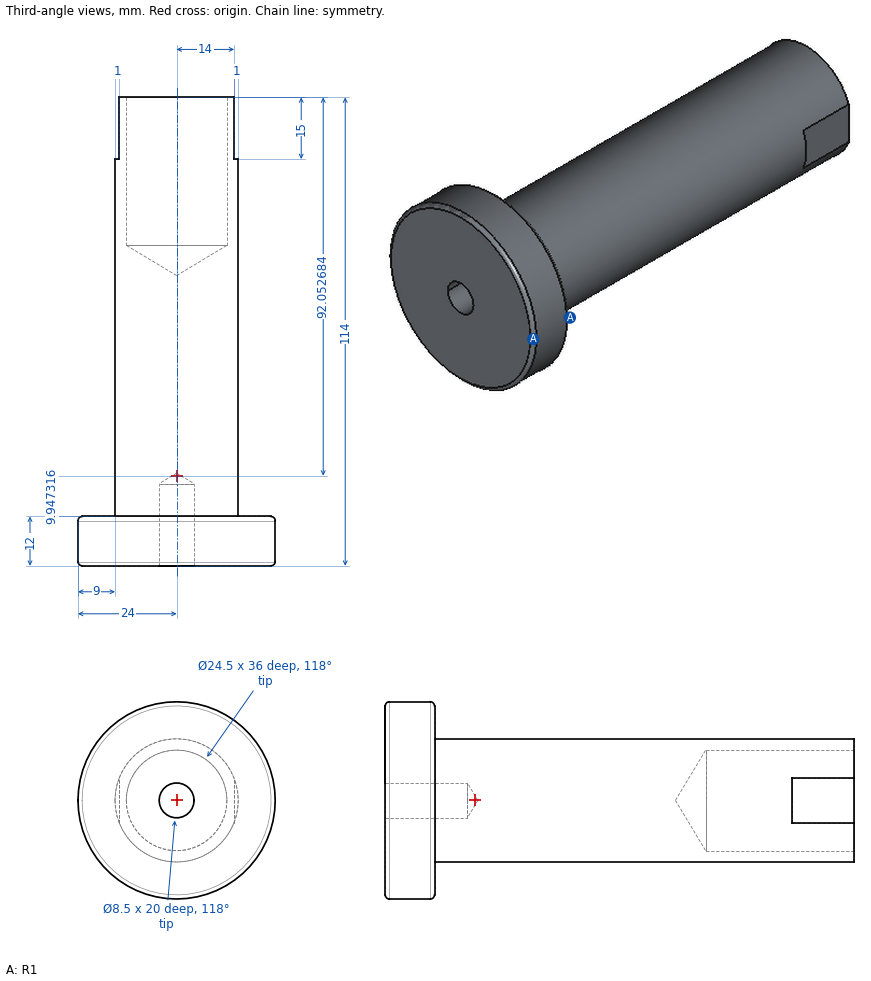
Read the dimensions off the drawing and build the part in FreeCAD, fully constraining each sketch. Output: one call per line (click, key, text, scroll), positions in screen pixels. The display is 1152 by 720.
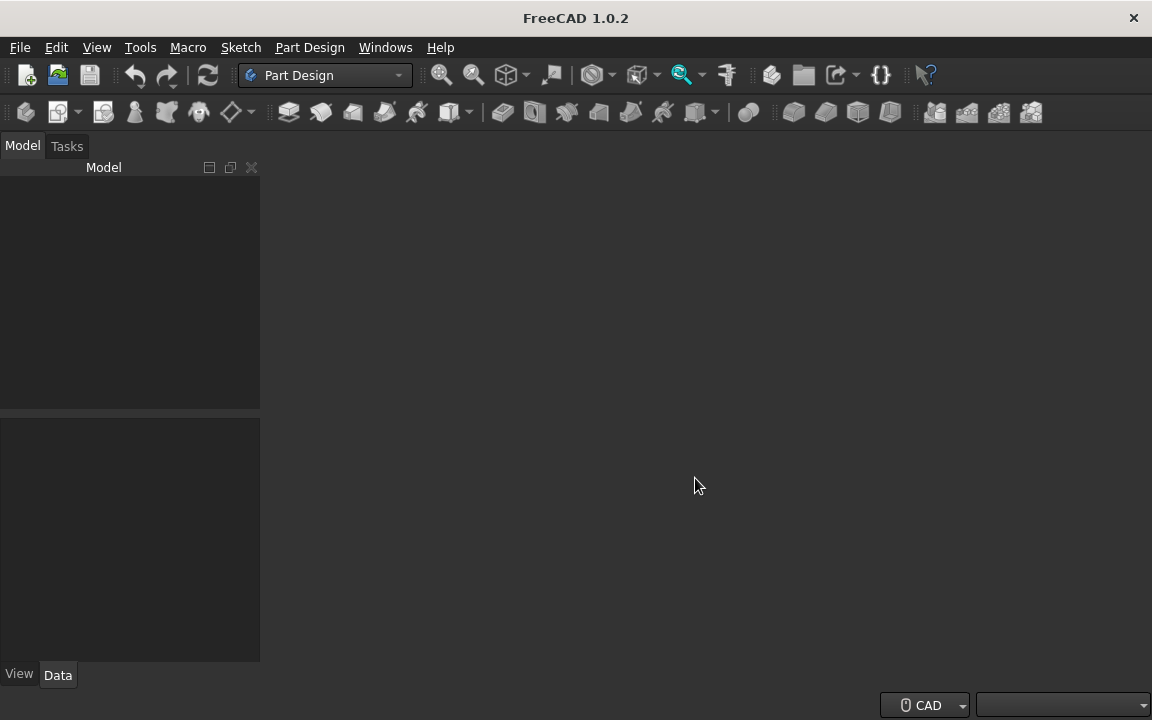
click(26, 76)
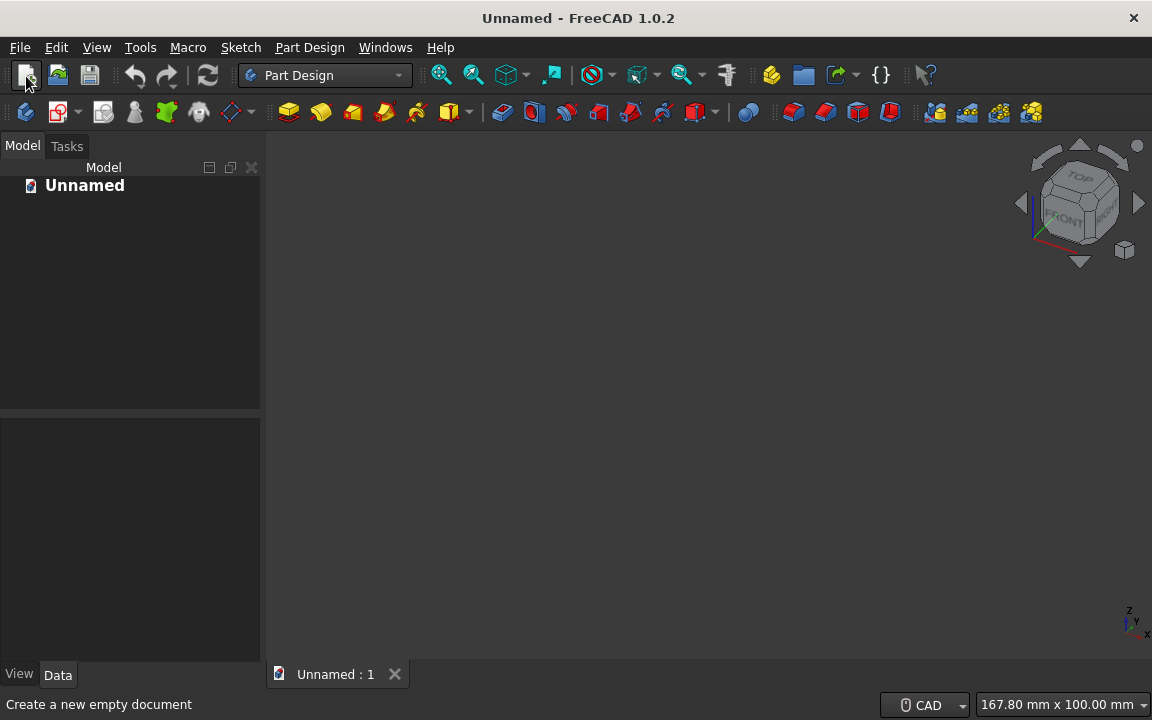
click(58, 112)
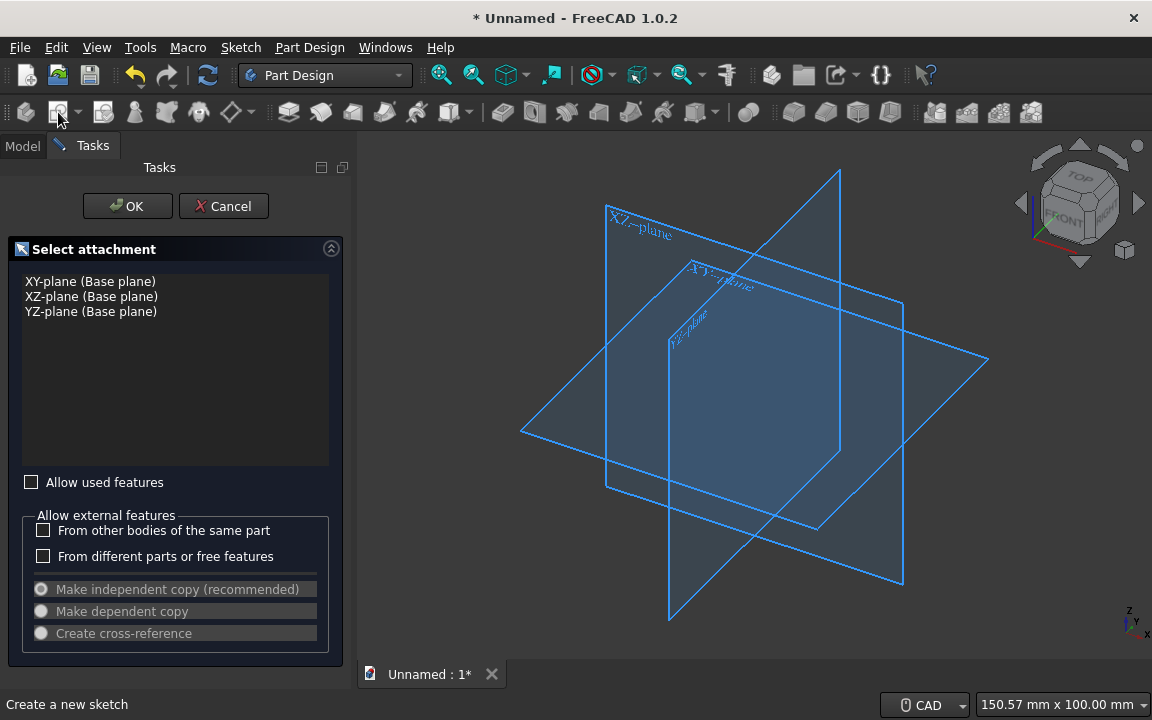
click(82, 282)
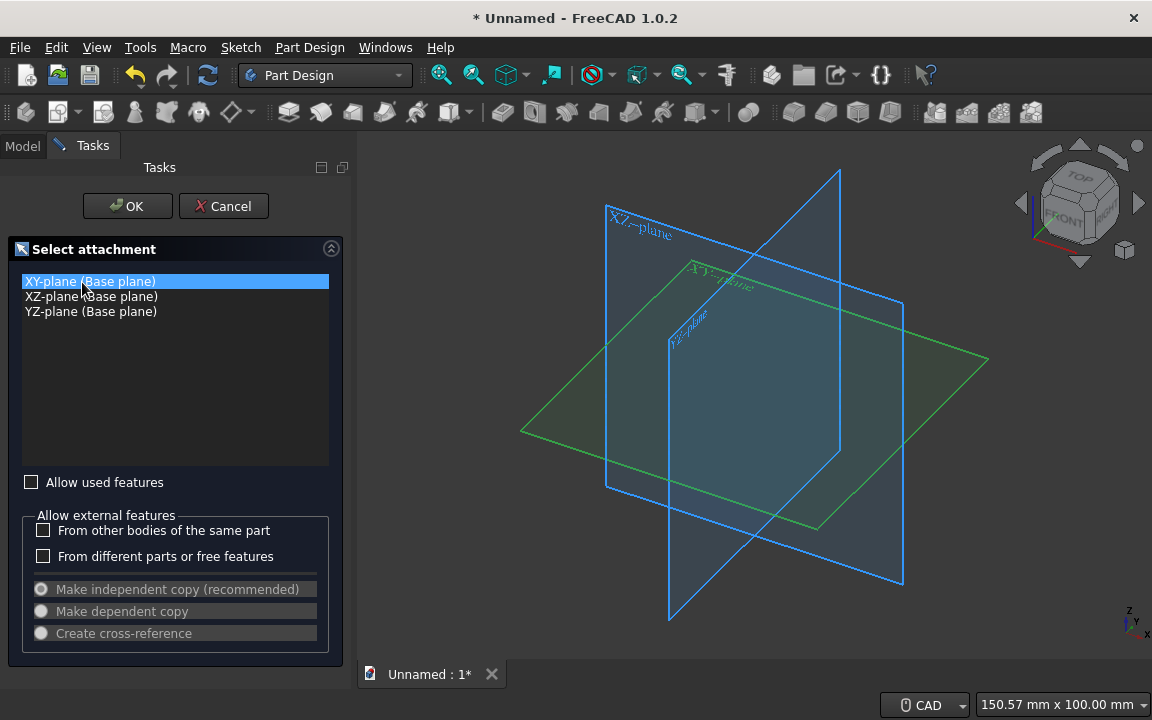
click(128, 206)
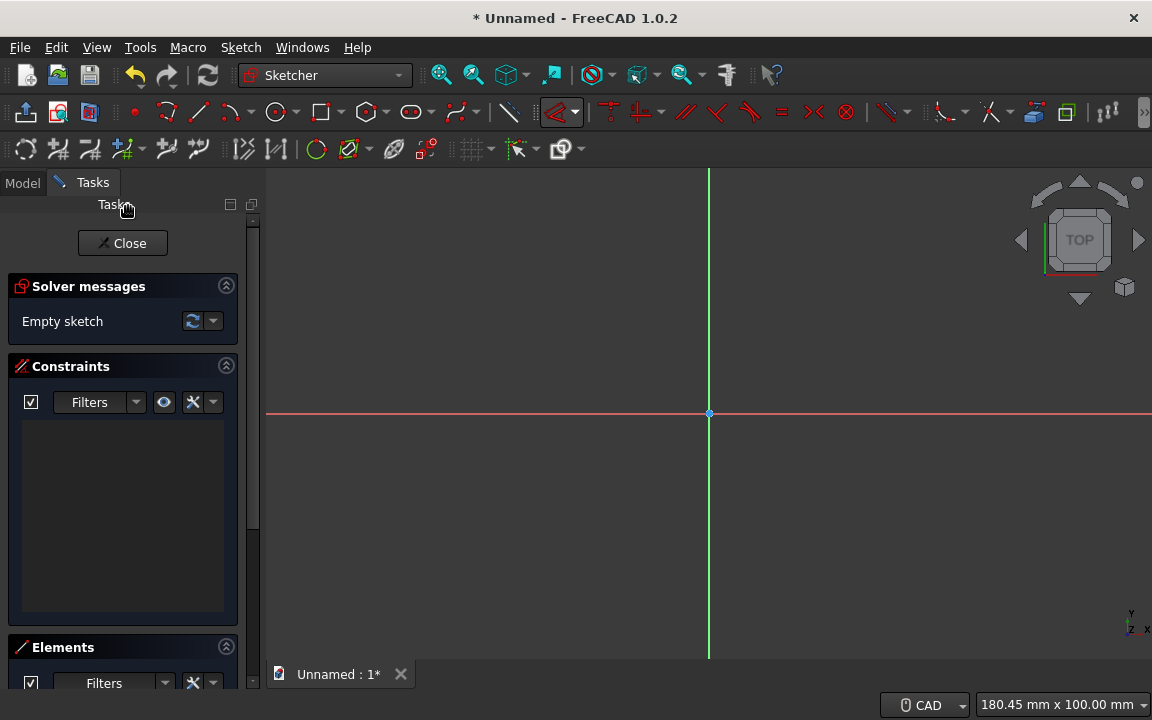
scroll(629, 623, down, 3)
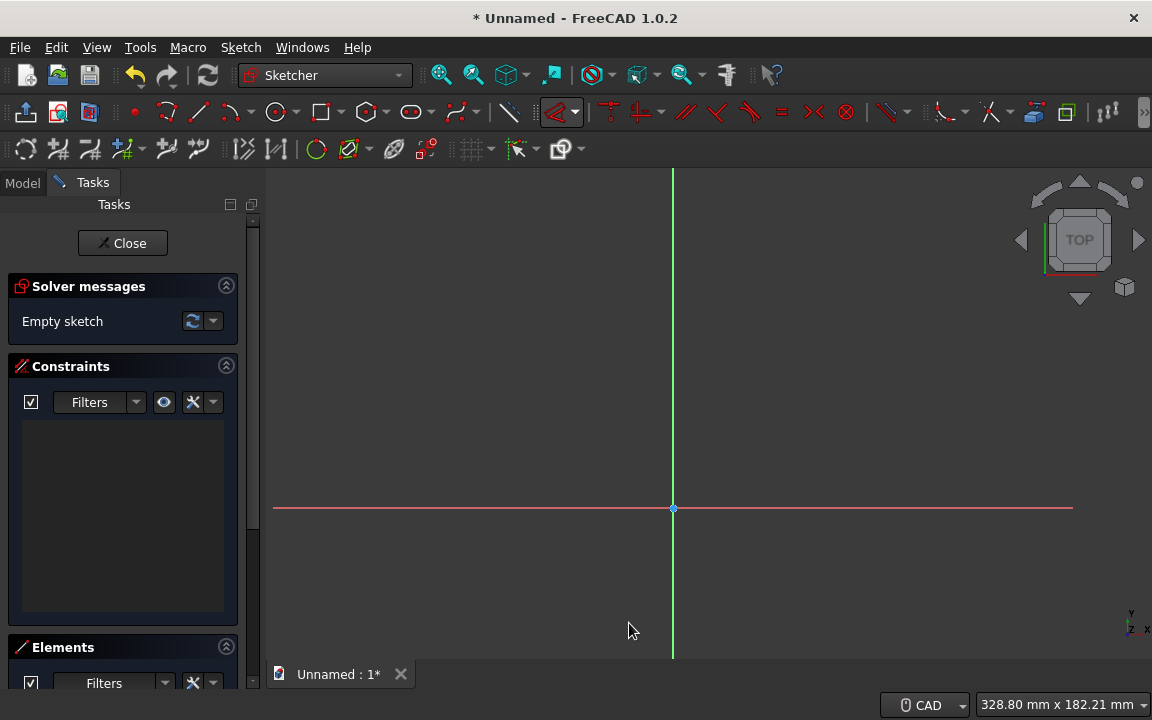
key(g)
key(m)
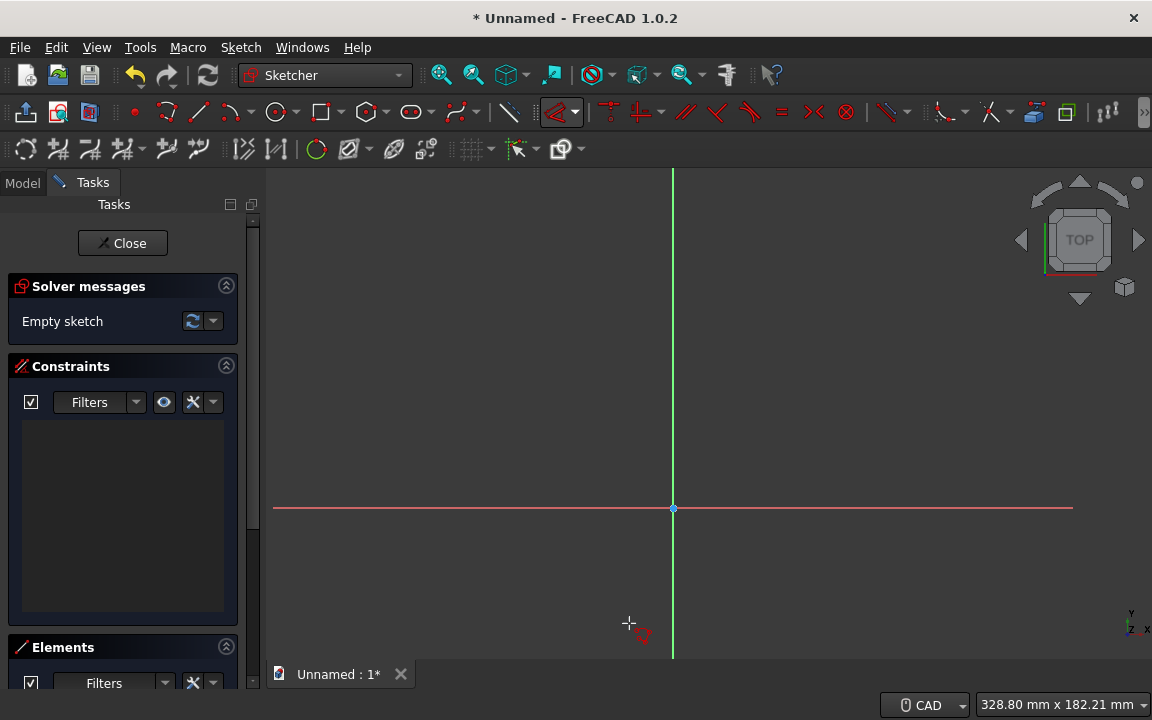
click(633, 535)
click(608, 535)
click(608, 568)
click(673, 568)
click(664, 260)
click(633, 260)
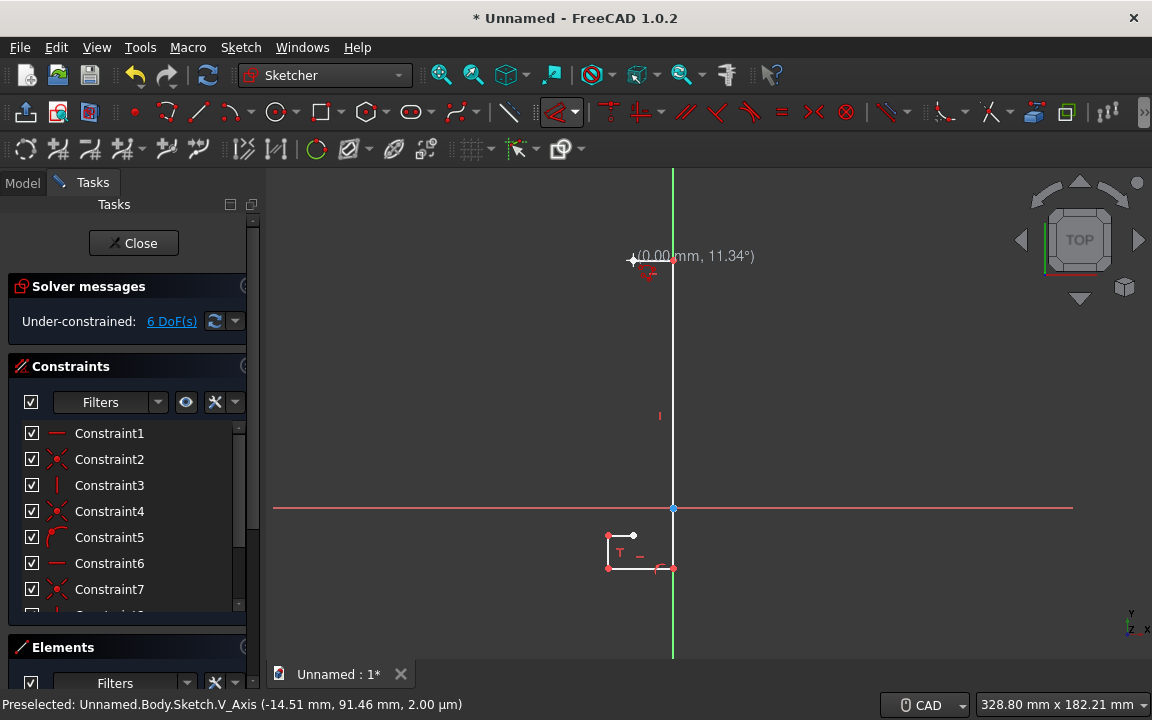
scroll(633, 535, up, 2)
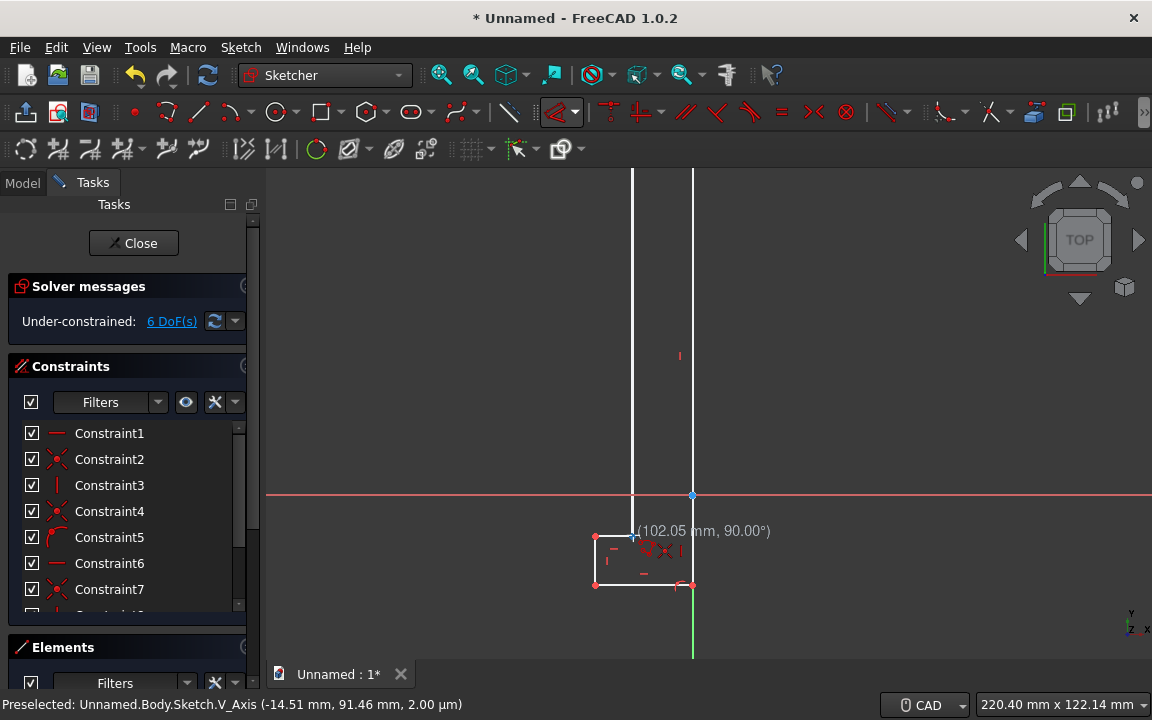
click(633, 536)
key(Escape)
key(Escape)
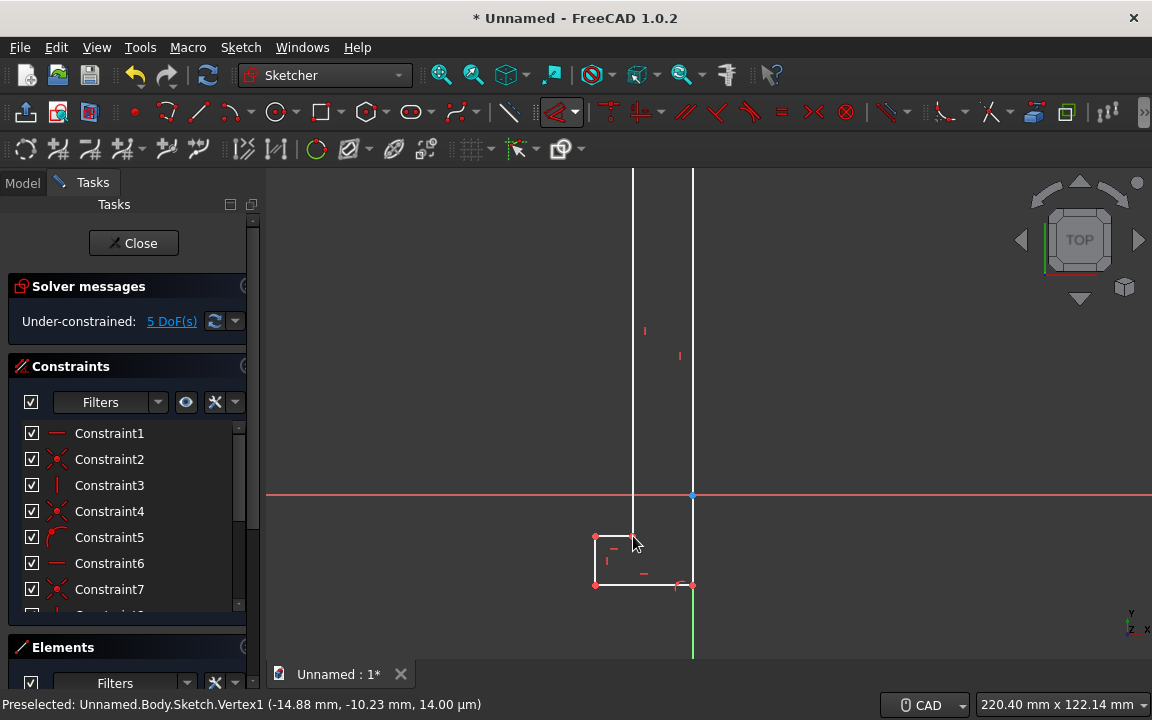
key(d)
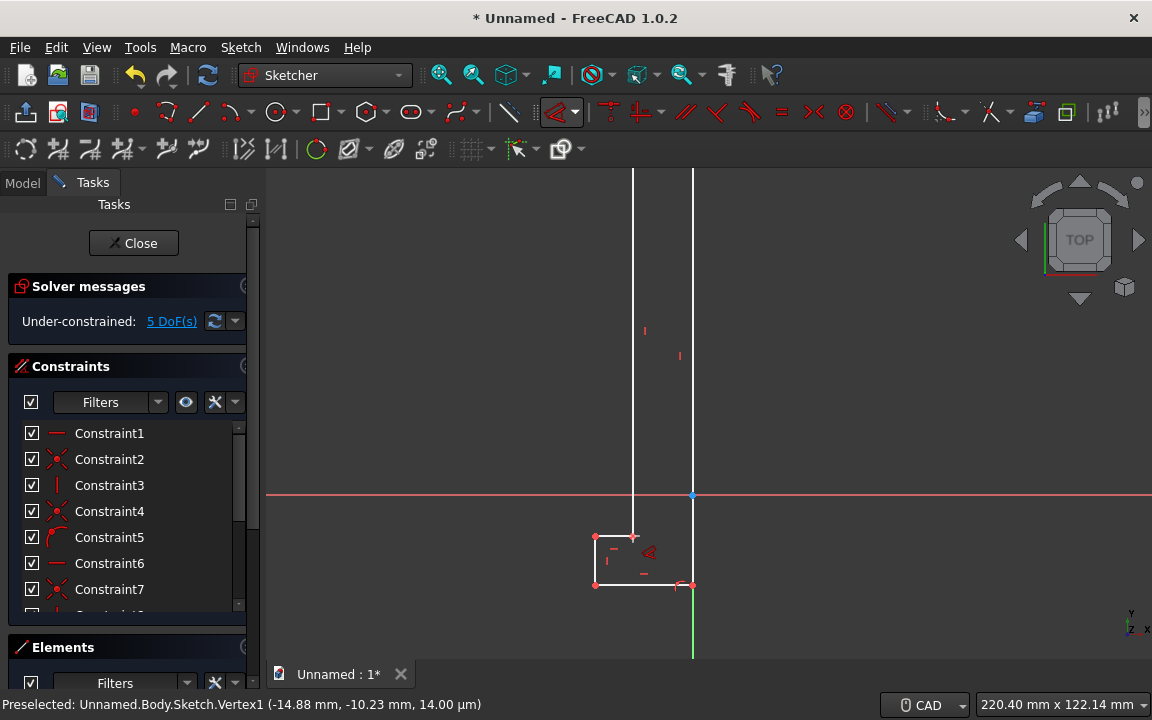
scroll(622, 536, up, 2)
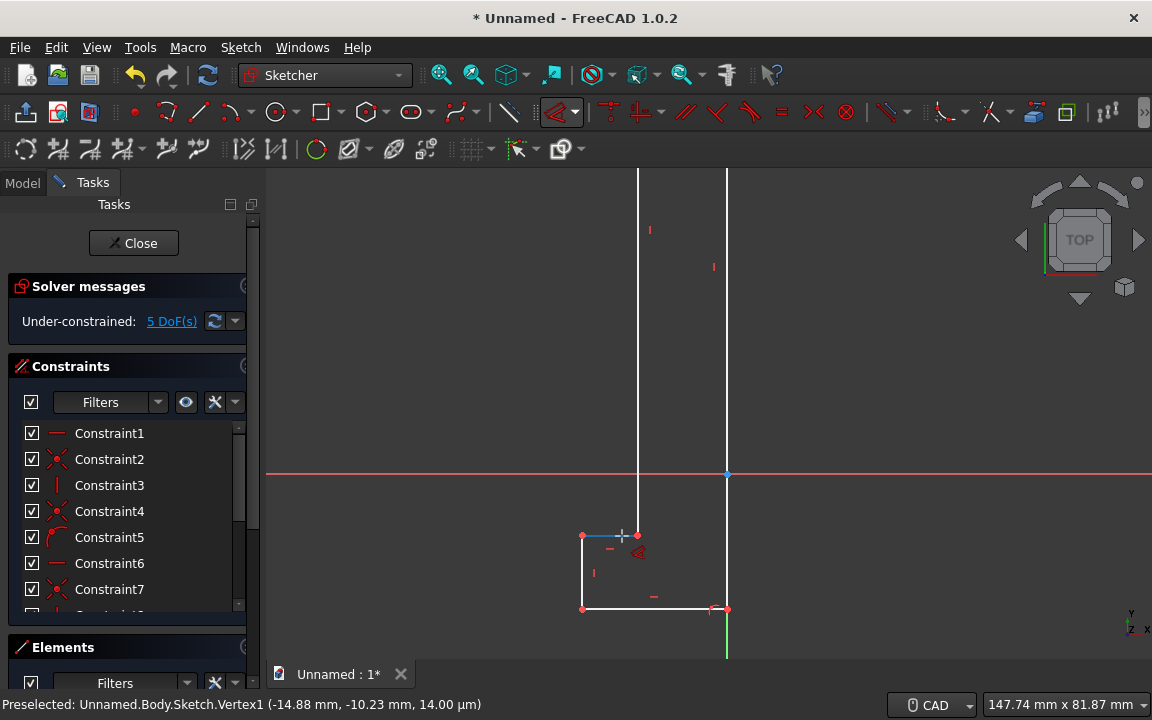
click(621, 536)
click(610, 570)